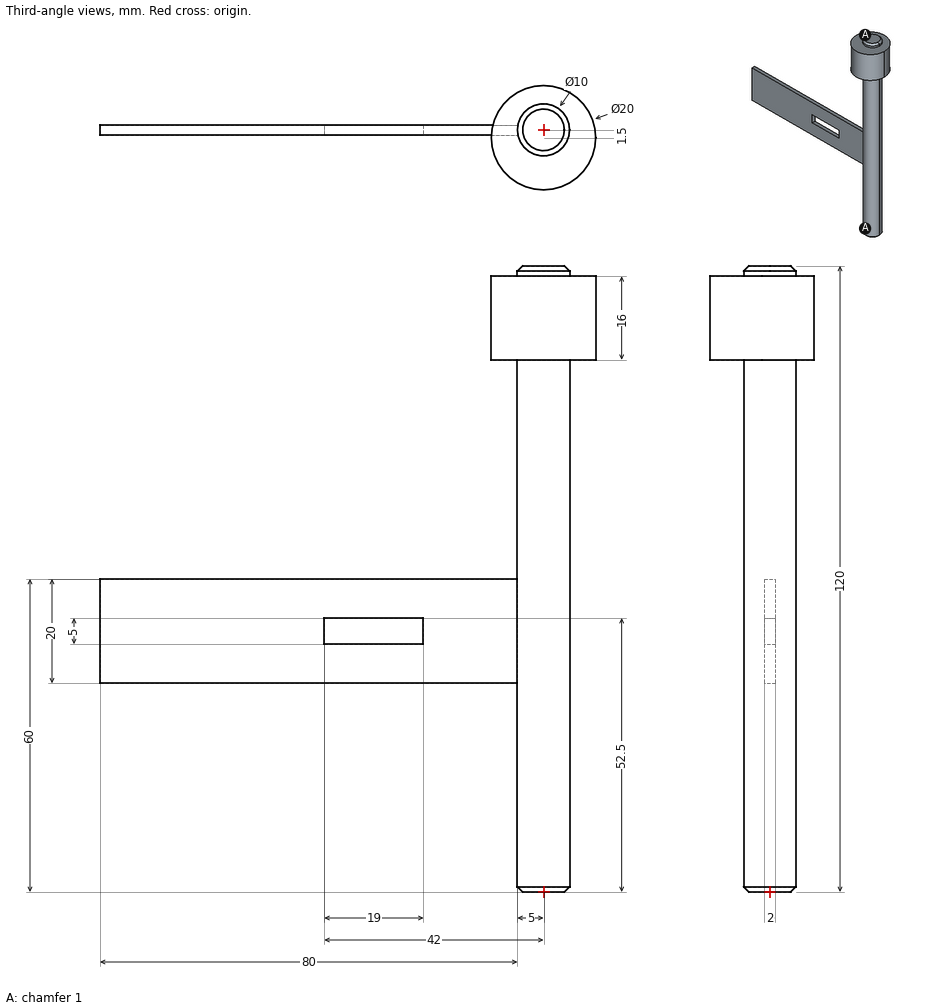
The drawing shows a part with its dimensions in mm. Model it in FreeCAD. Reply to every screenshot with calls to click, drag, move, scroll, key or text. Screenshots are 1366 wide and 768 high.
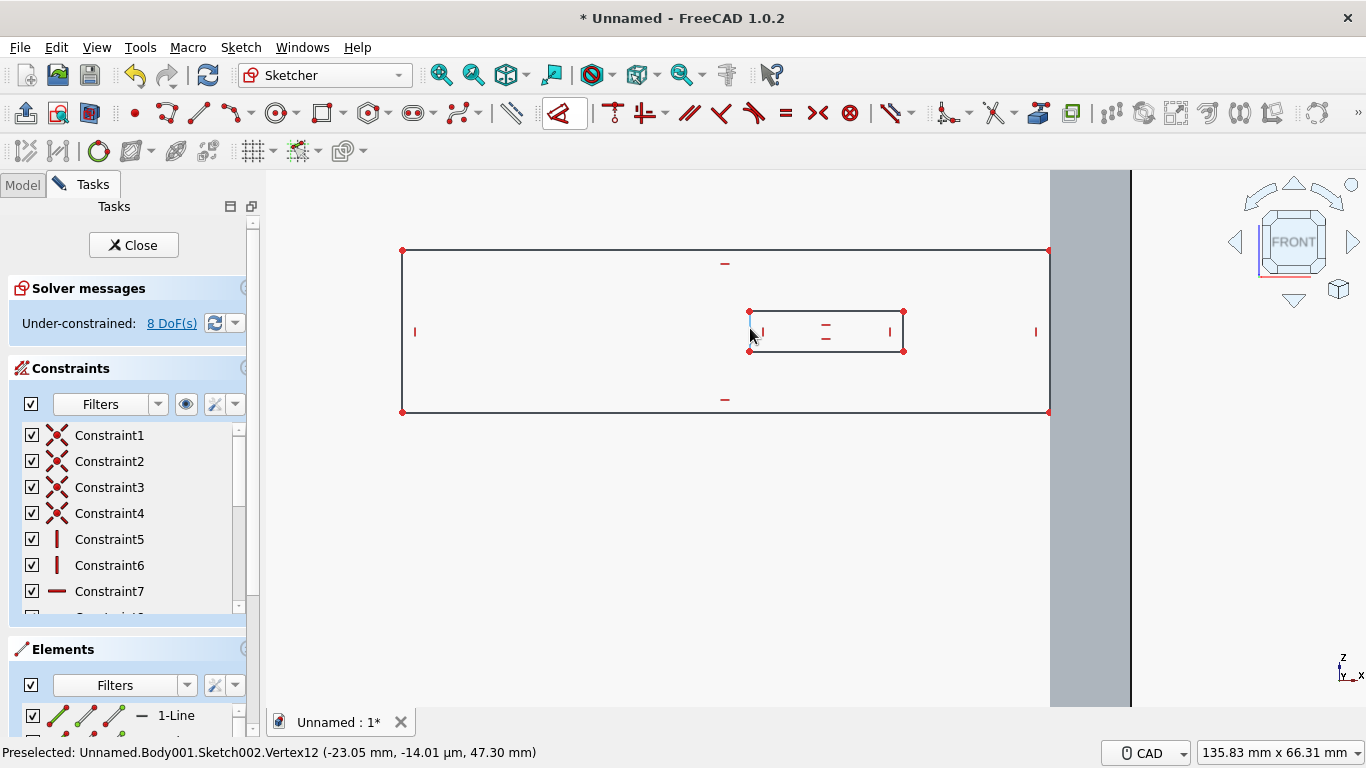
click(750, 328)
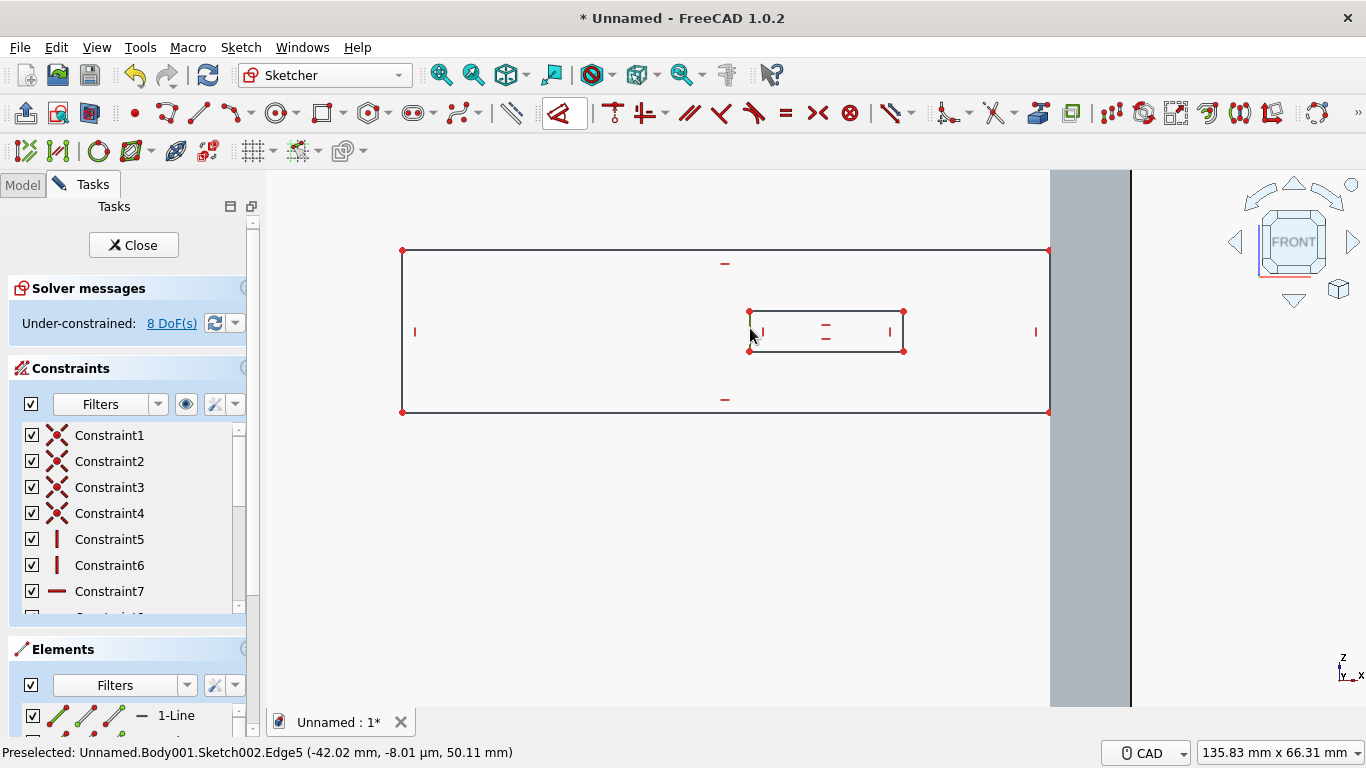
key(i)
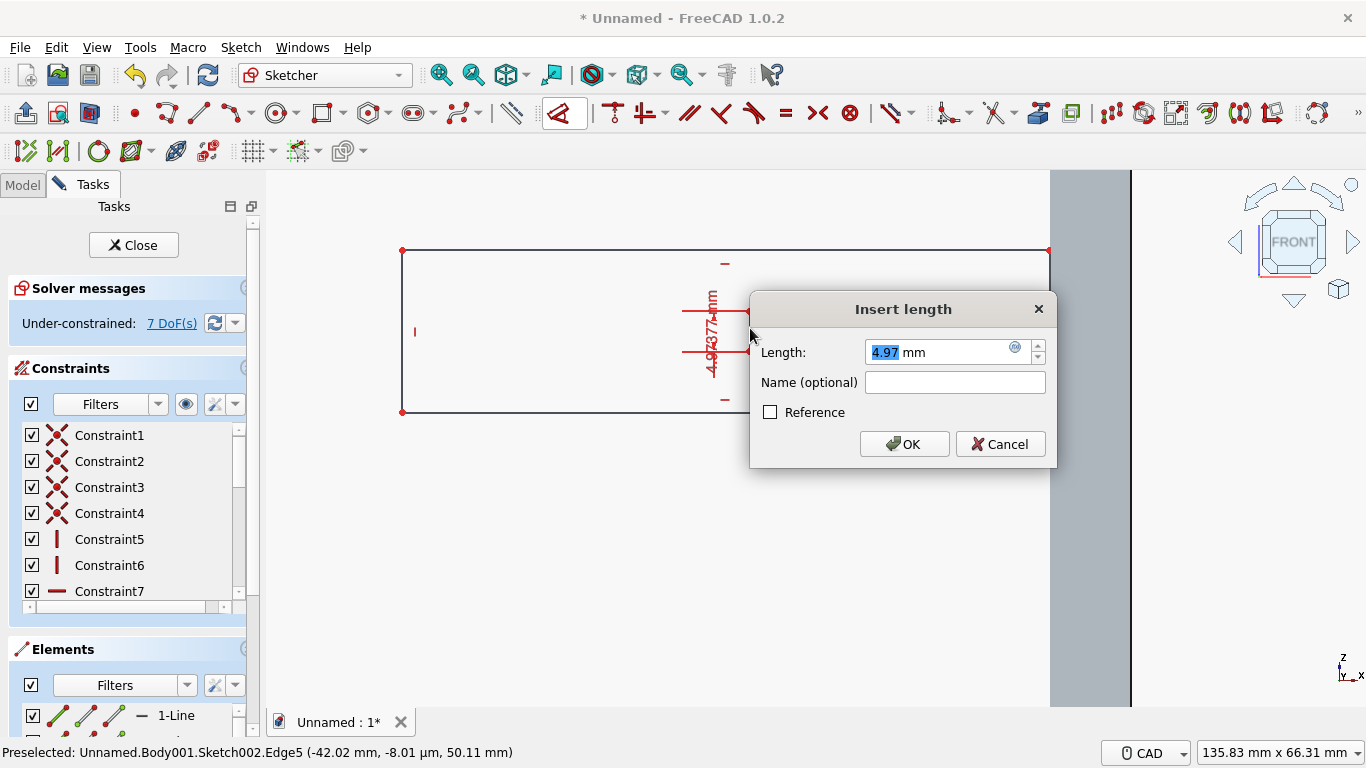
text(5)
key(Return)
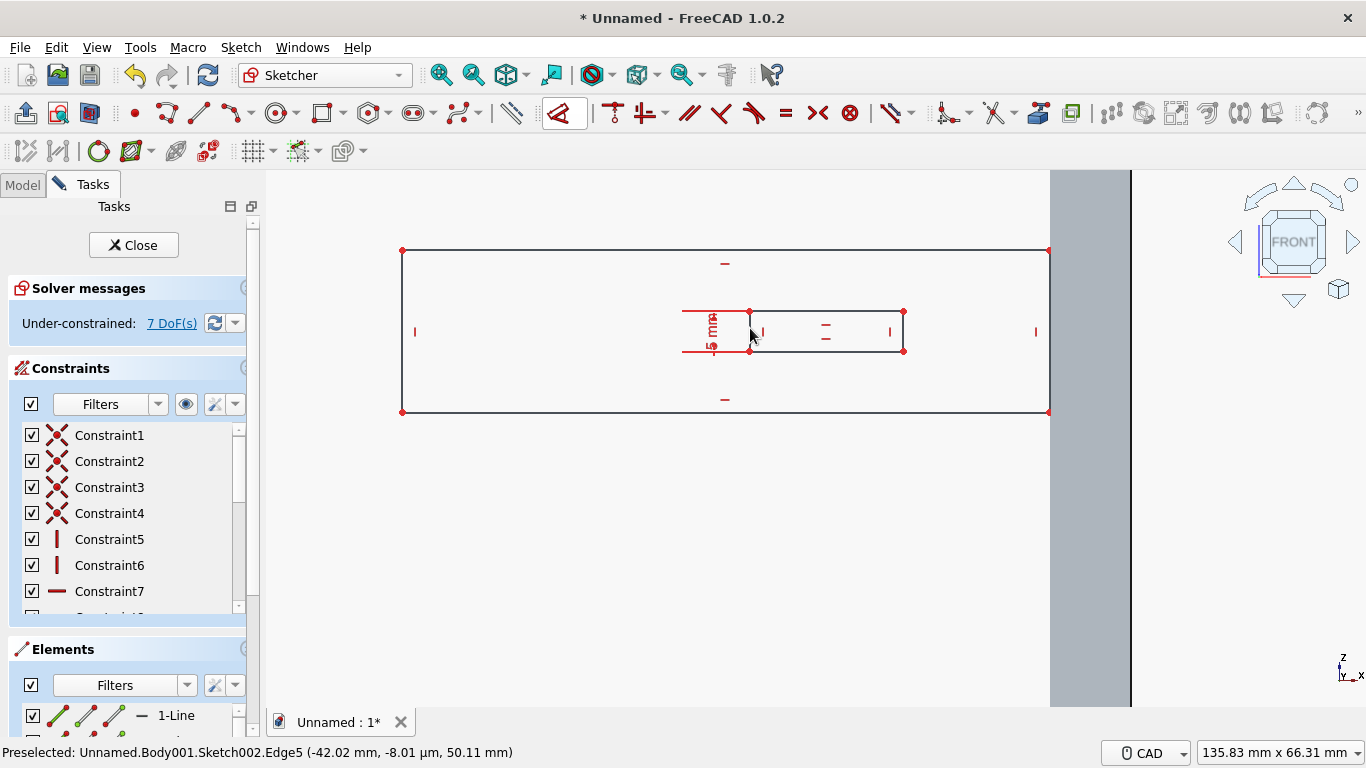
click(402, 299)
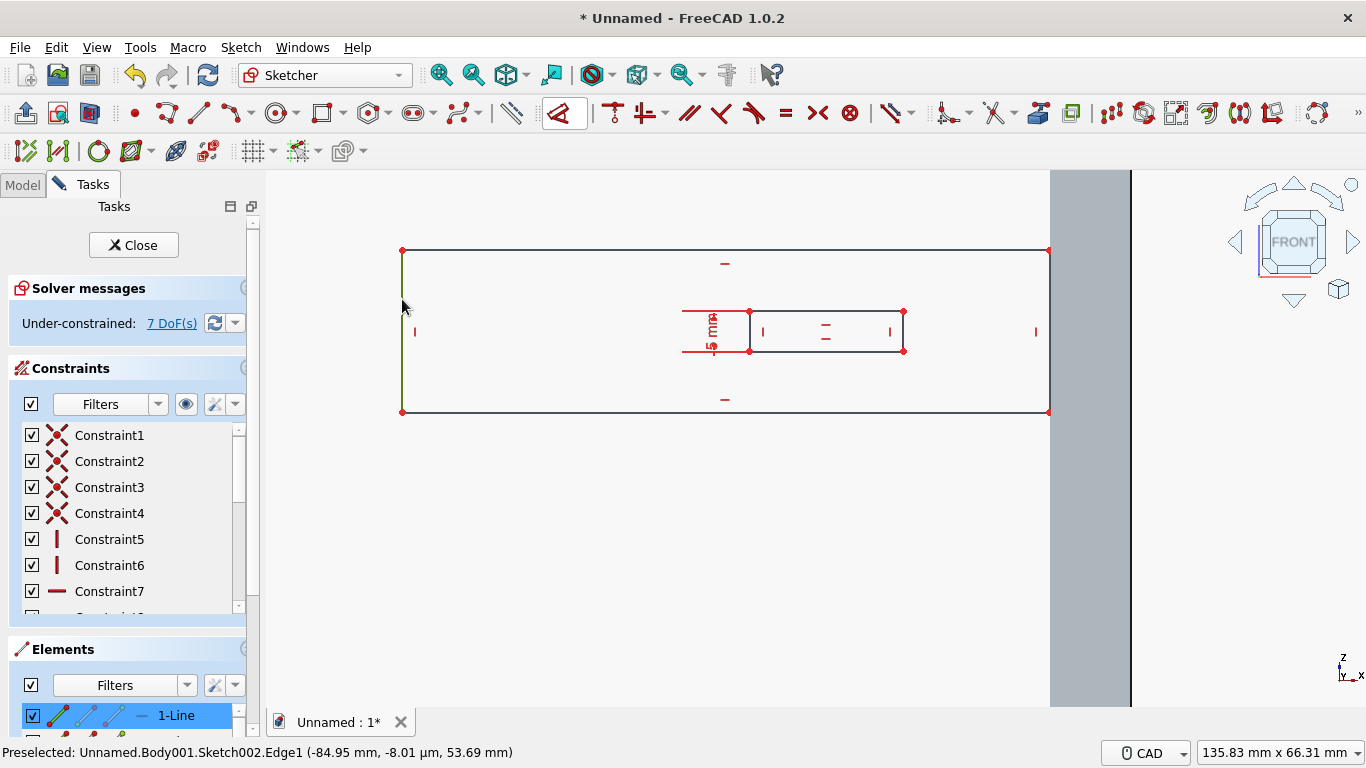
click(582, 114)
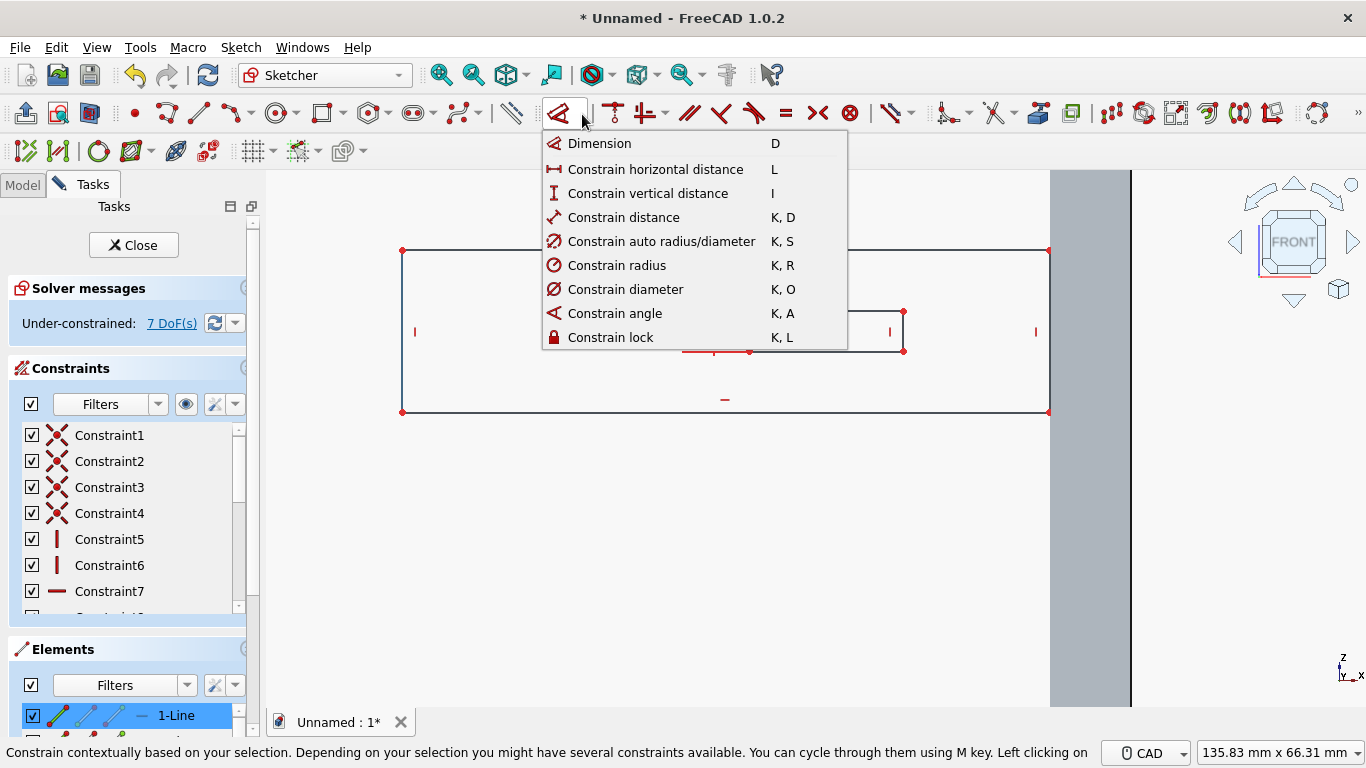
click(695, 193)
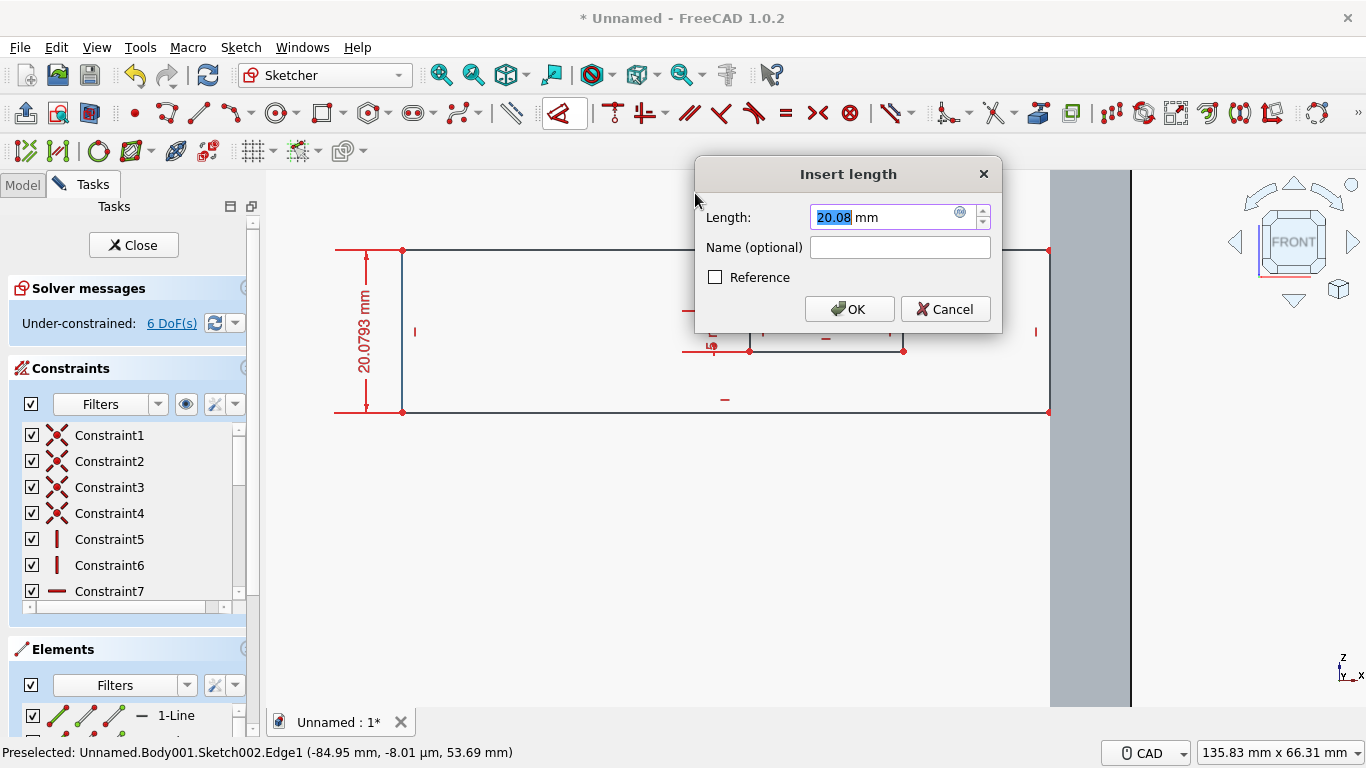
text(20)
key(Return)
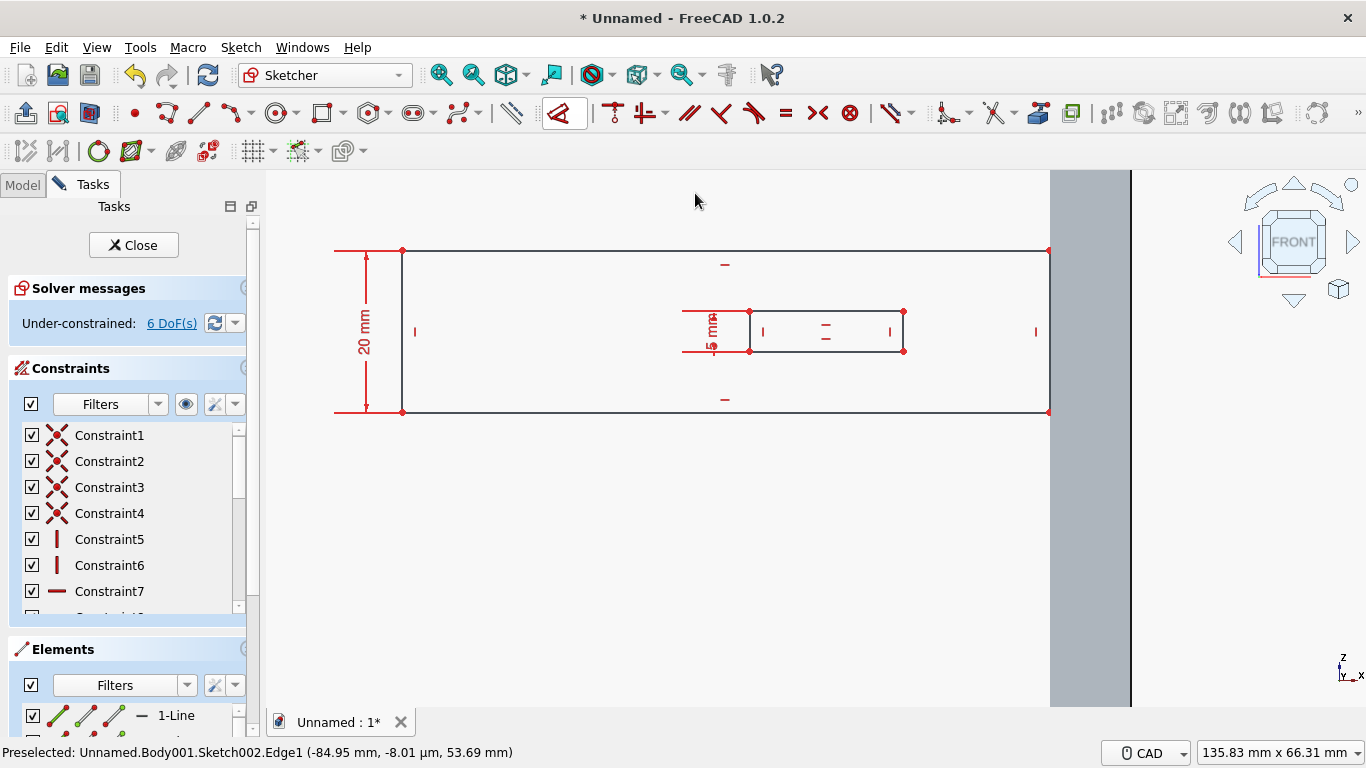
click(596, 413)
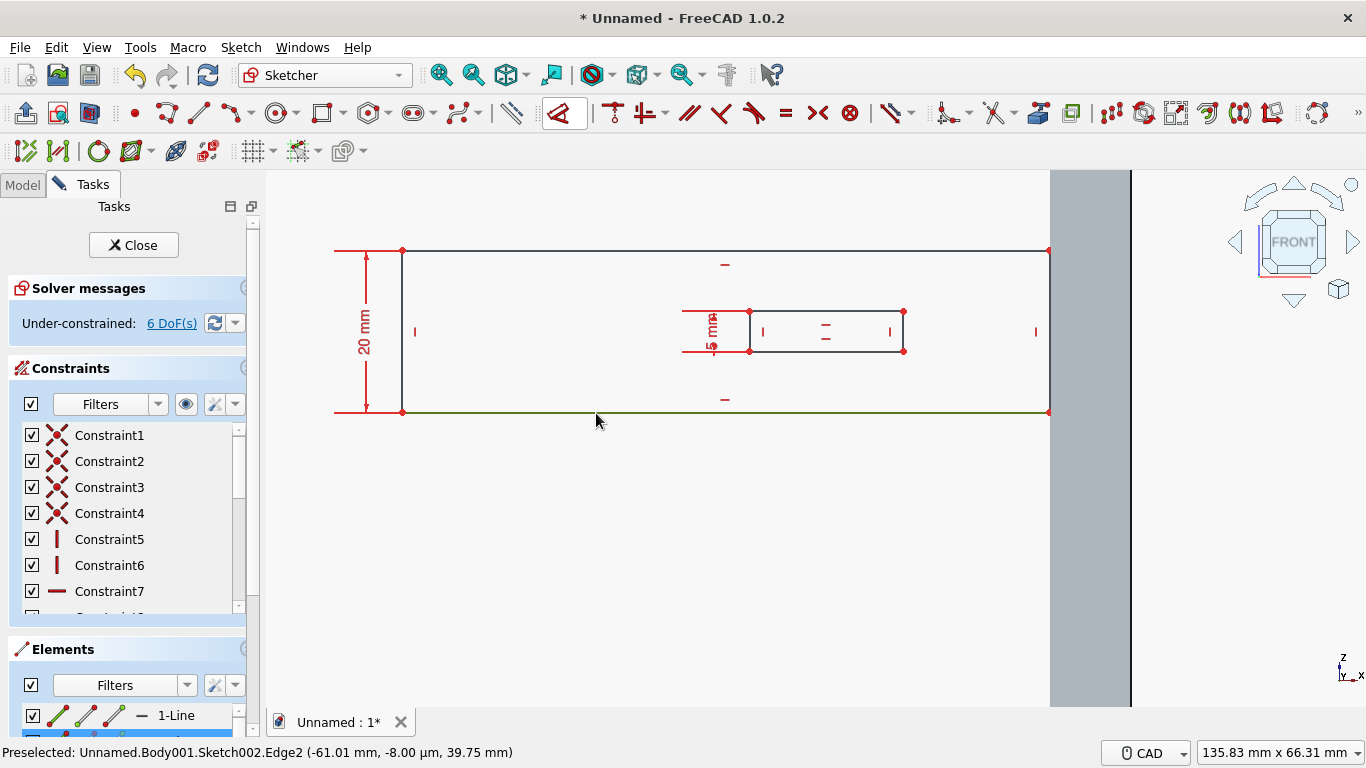
click(582, 114)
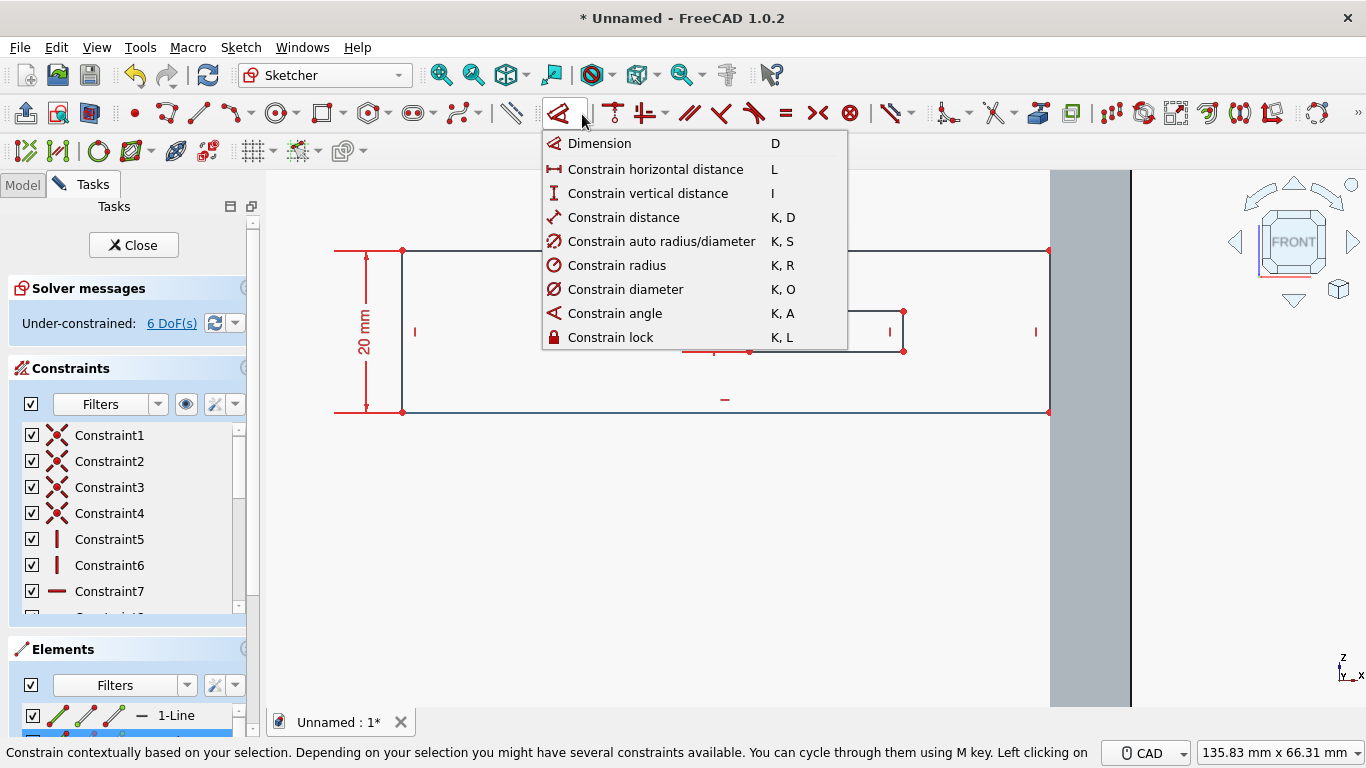
click(695, 169)